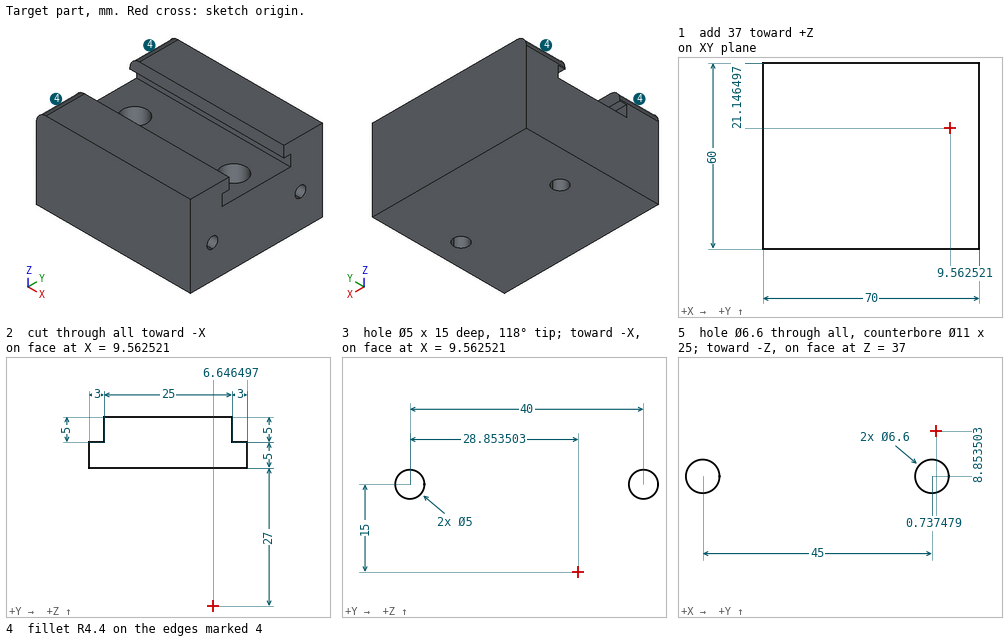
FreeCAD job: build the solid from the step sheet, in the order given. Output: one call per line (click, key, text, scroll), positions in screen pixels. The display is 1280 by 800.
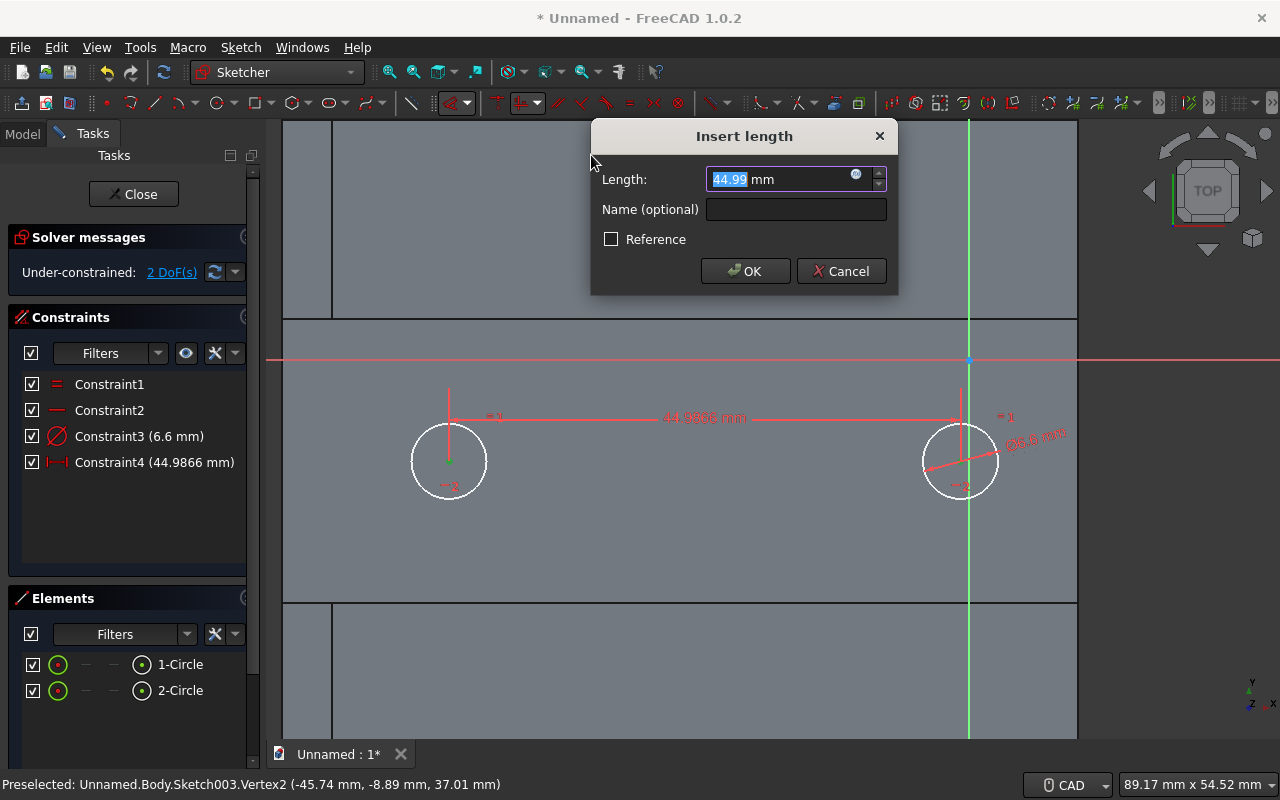
text(45)
key(Return)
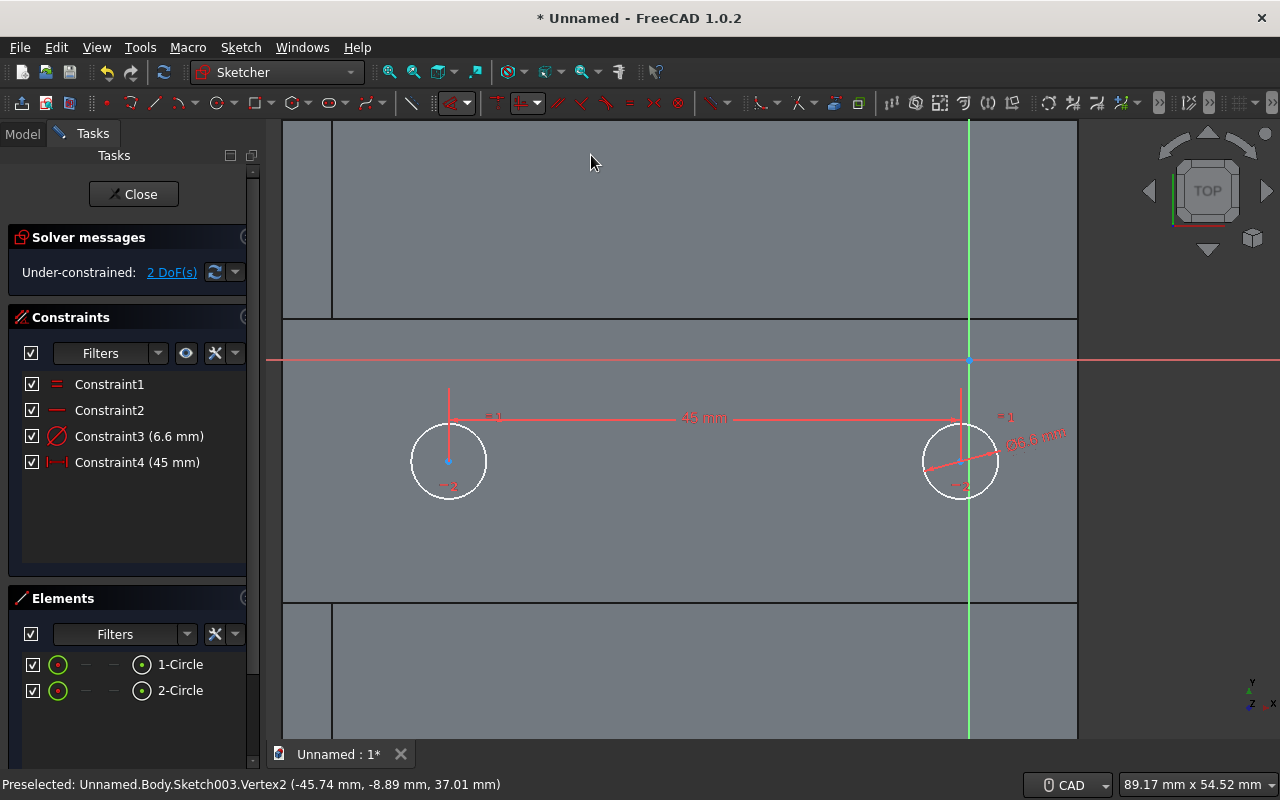
scroll(961, 461, up, 8)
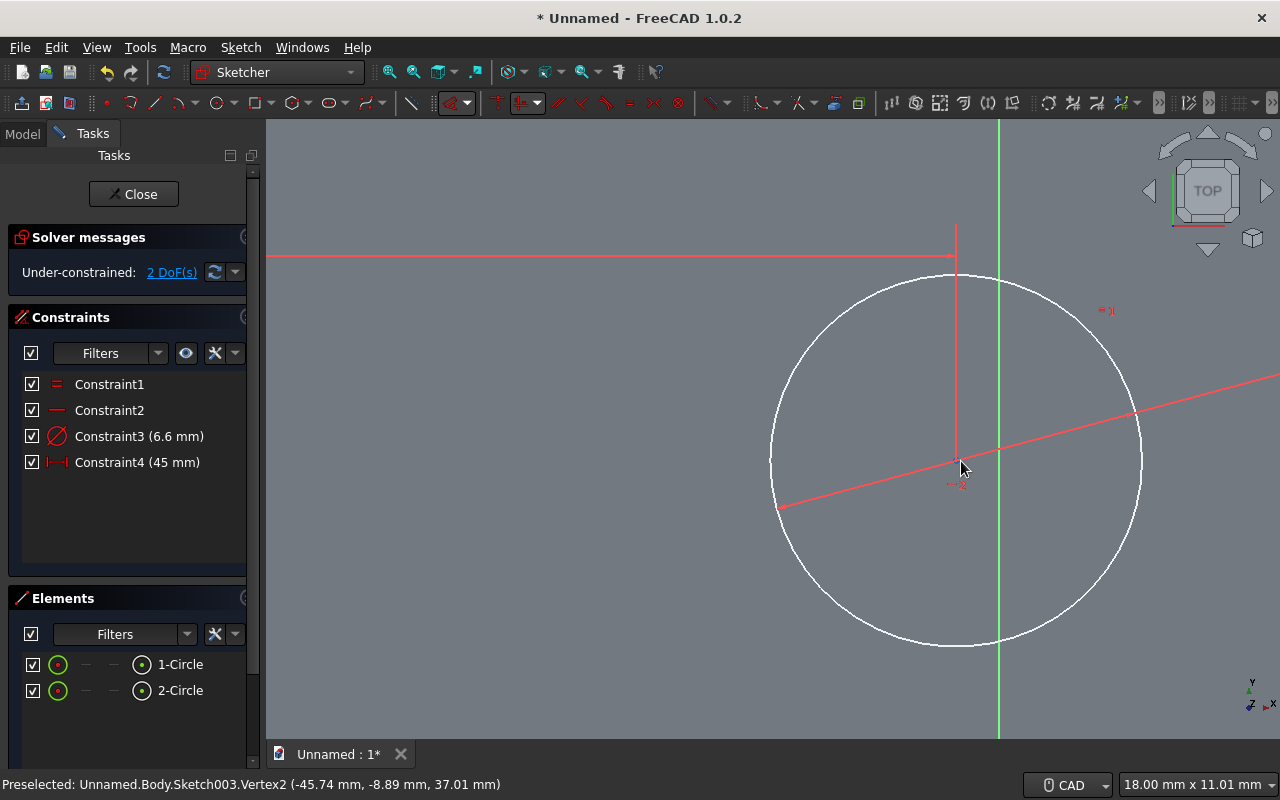
click(956, 461)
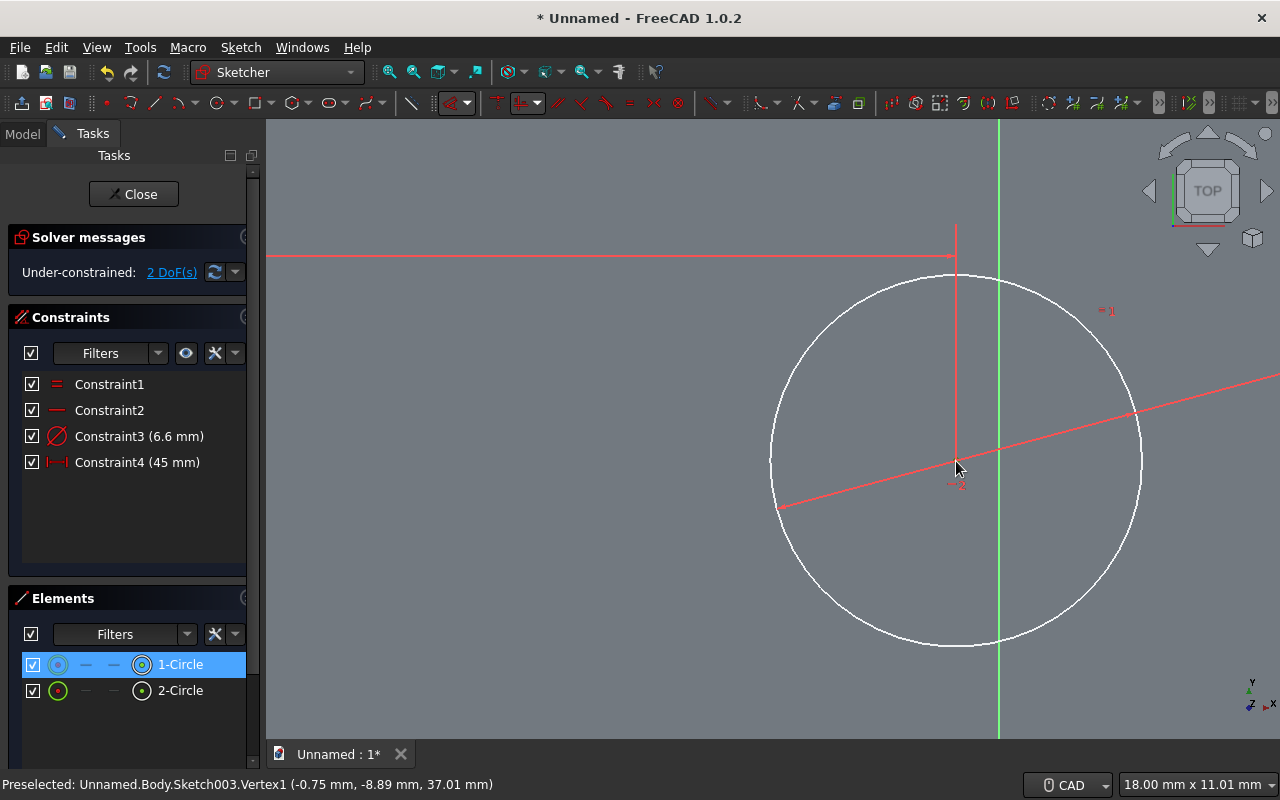
click(470, 104)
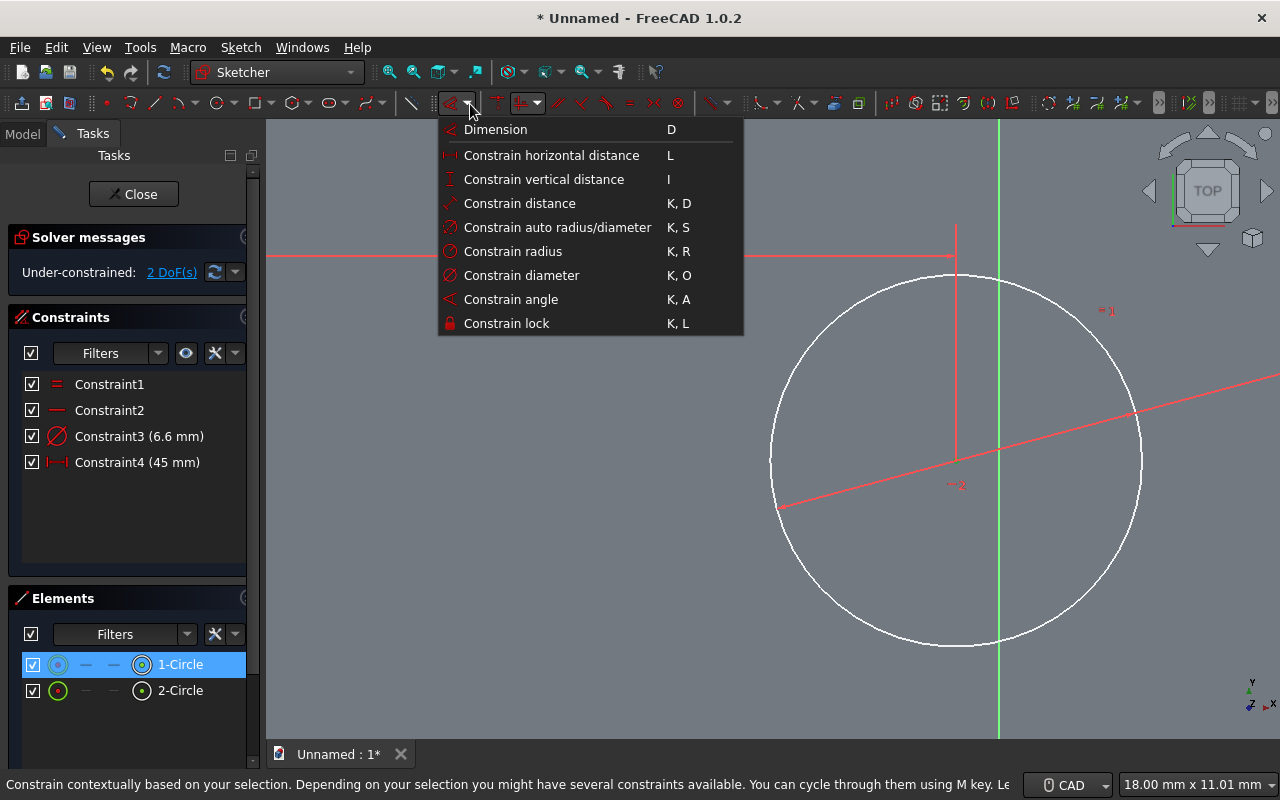
click(591, 155)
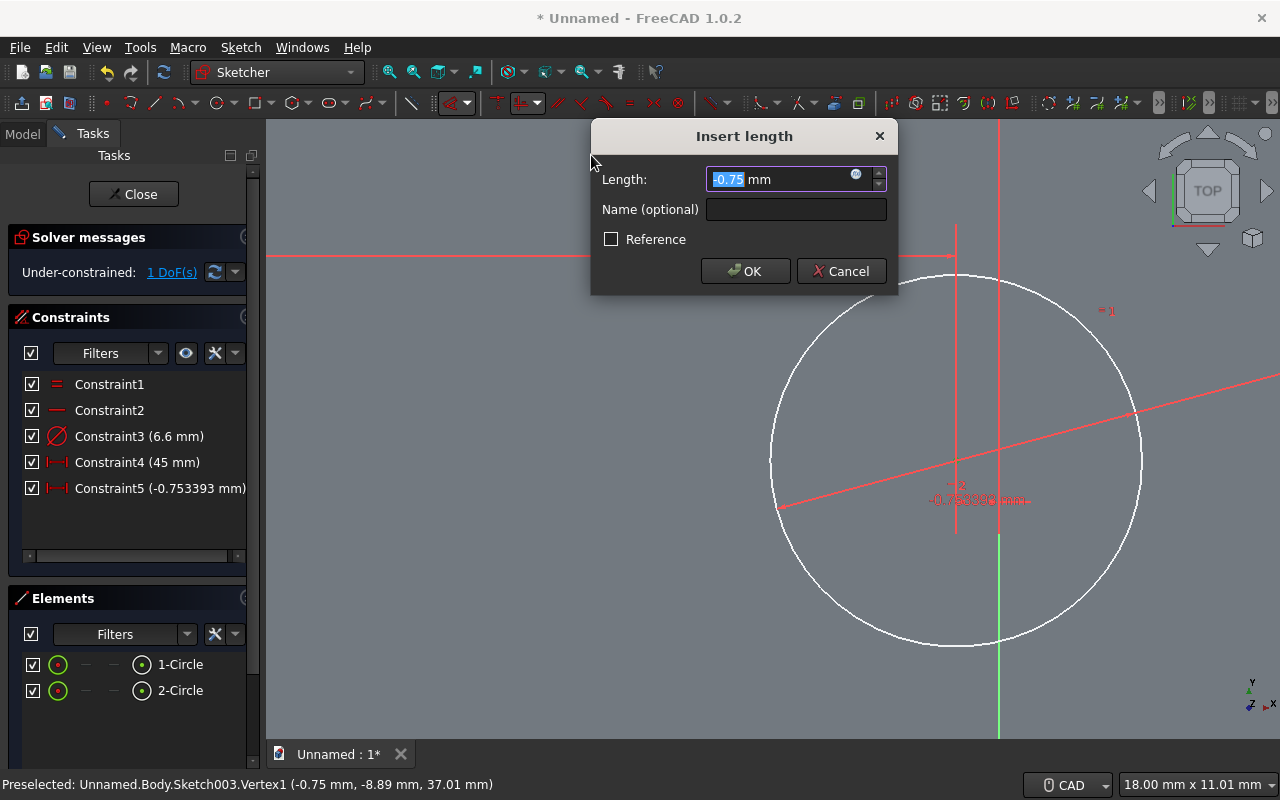
text(-0.737479)
key(Return)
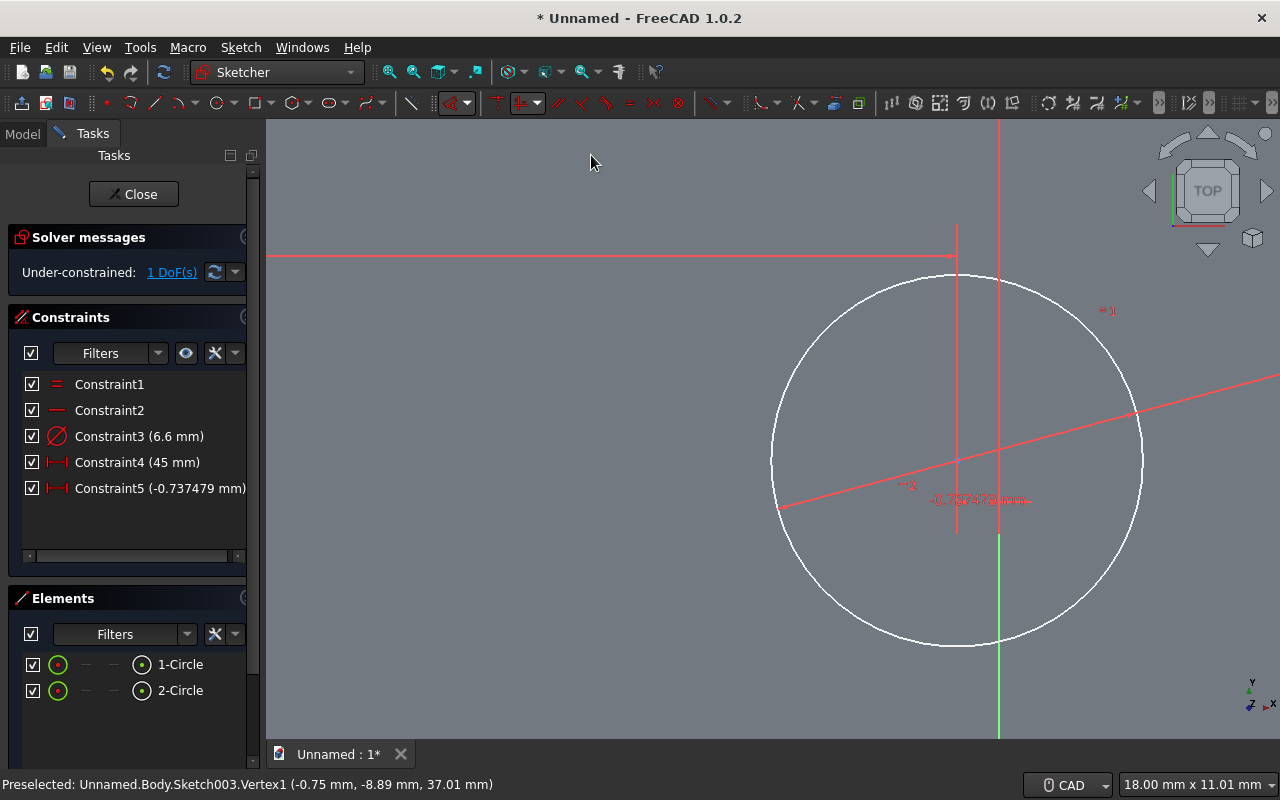
scroll(961, 461, down, 8)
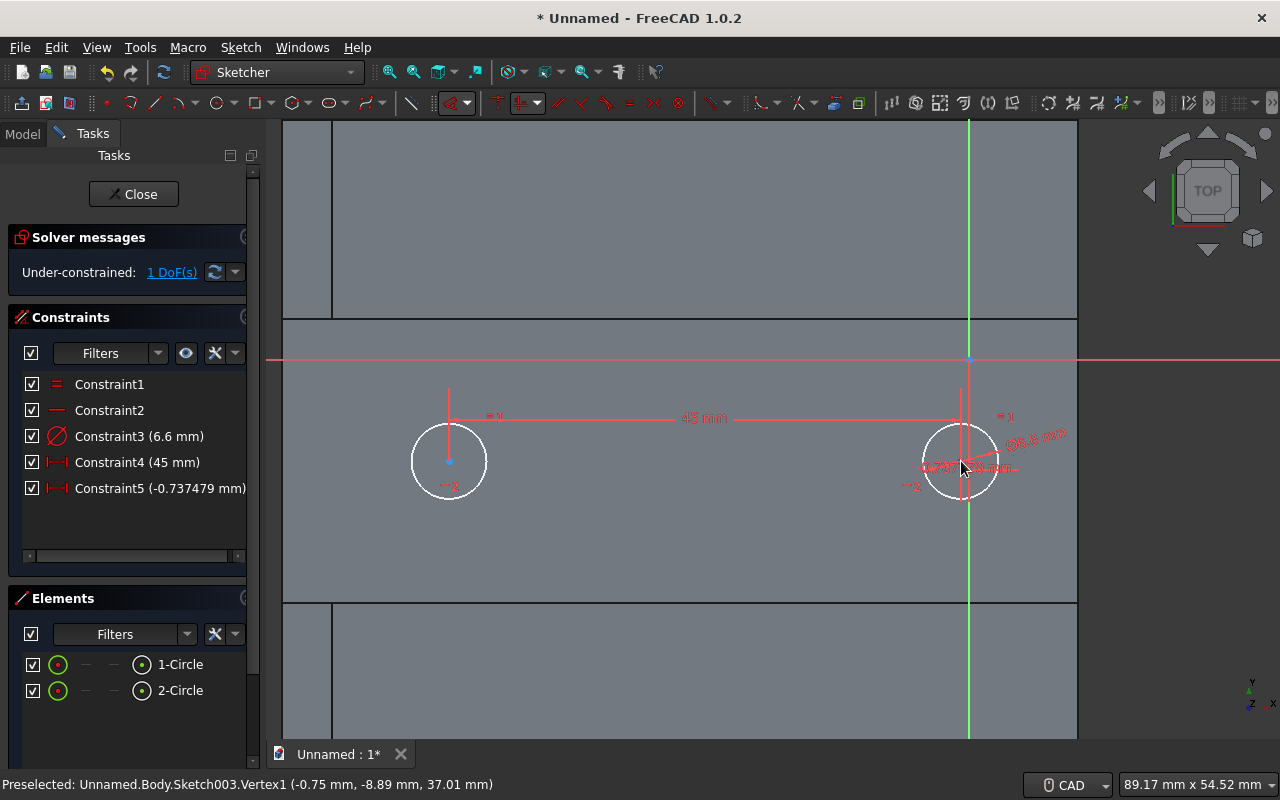
click(961, 461)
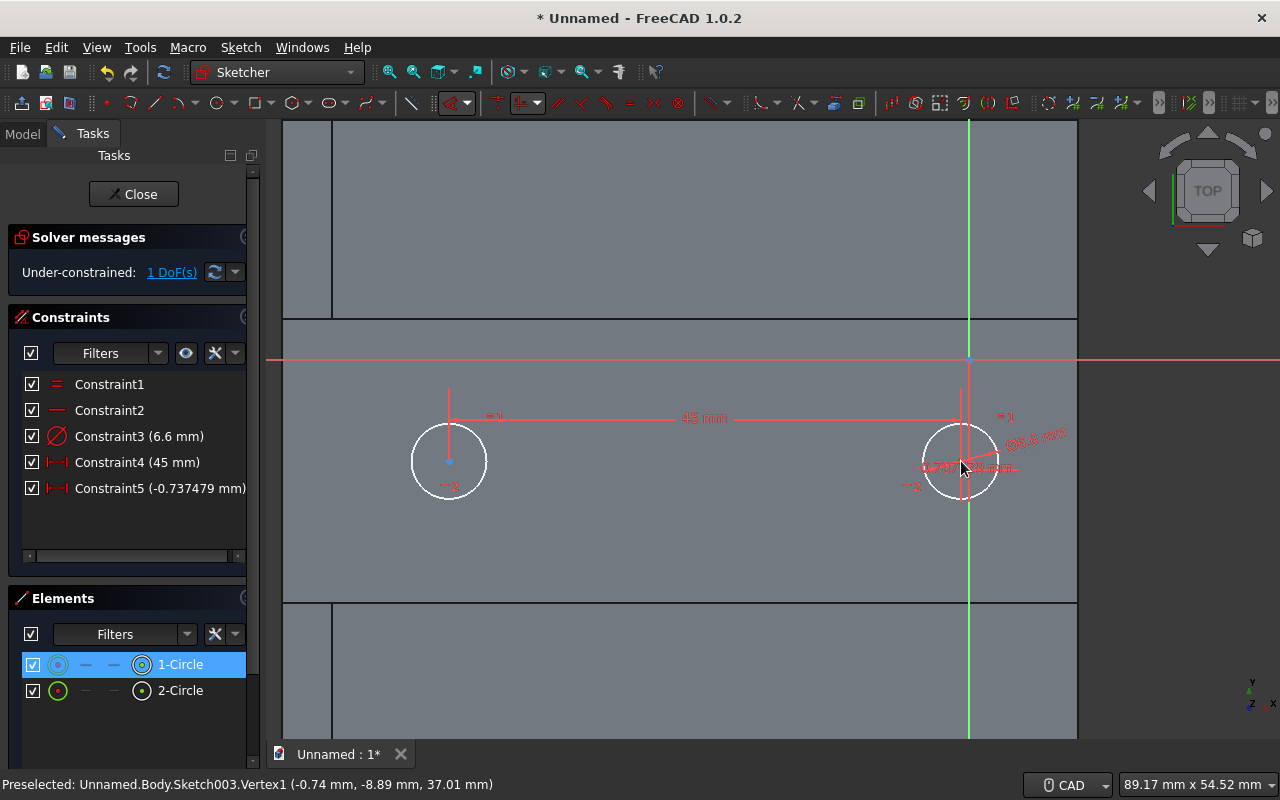
key(i)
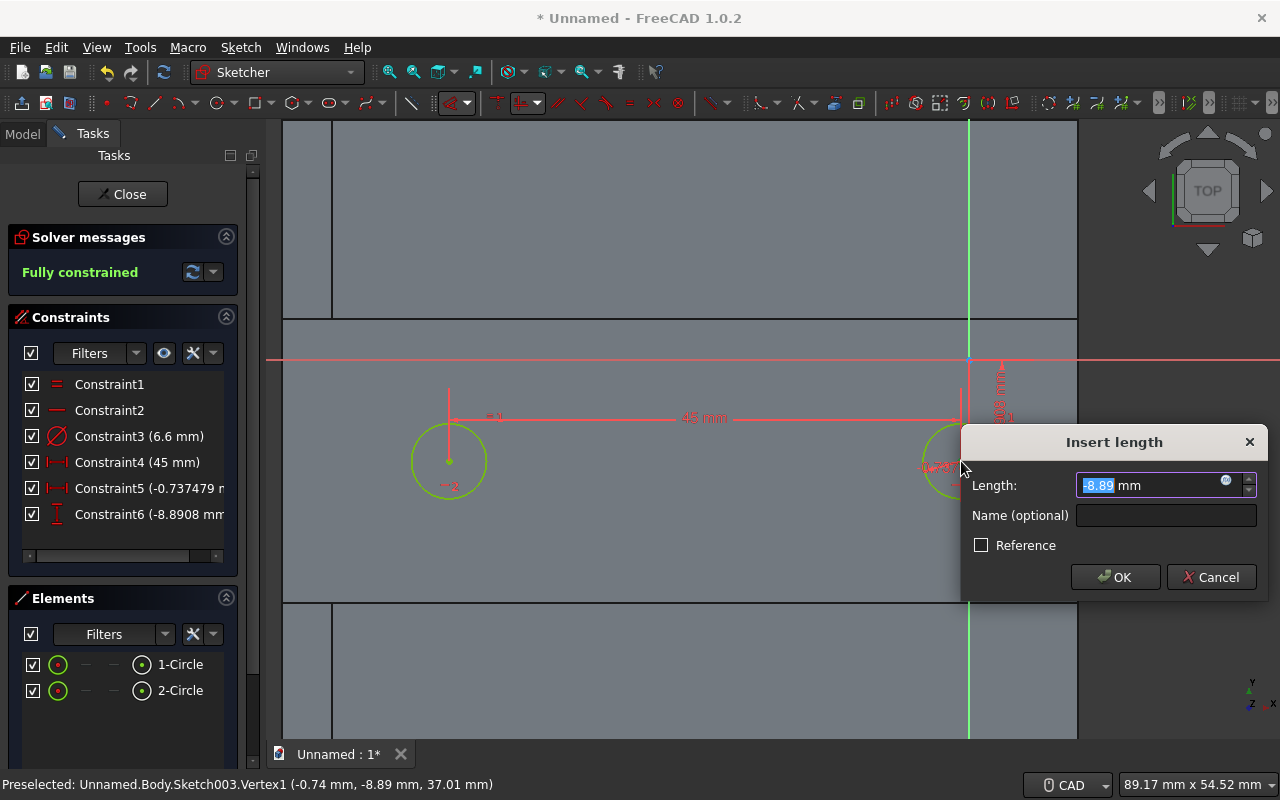
text(-8.853503)
key(Return)